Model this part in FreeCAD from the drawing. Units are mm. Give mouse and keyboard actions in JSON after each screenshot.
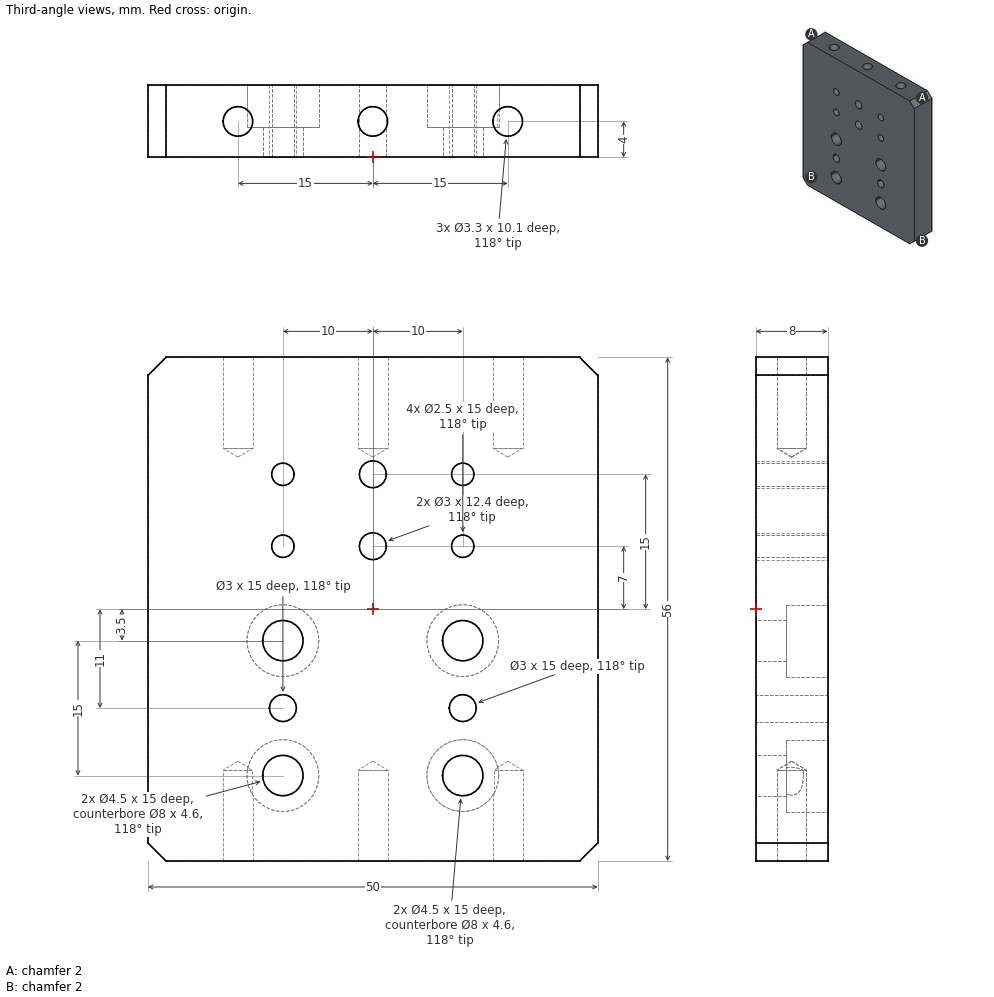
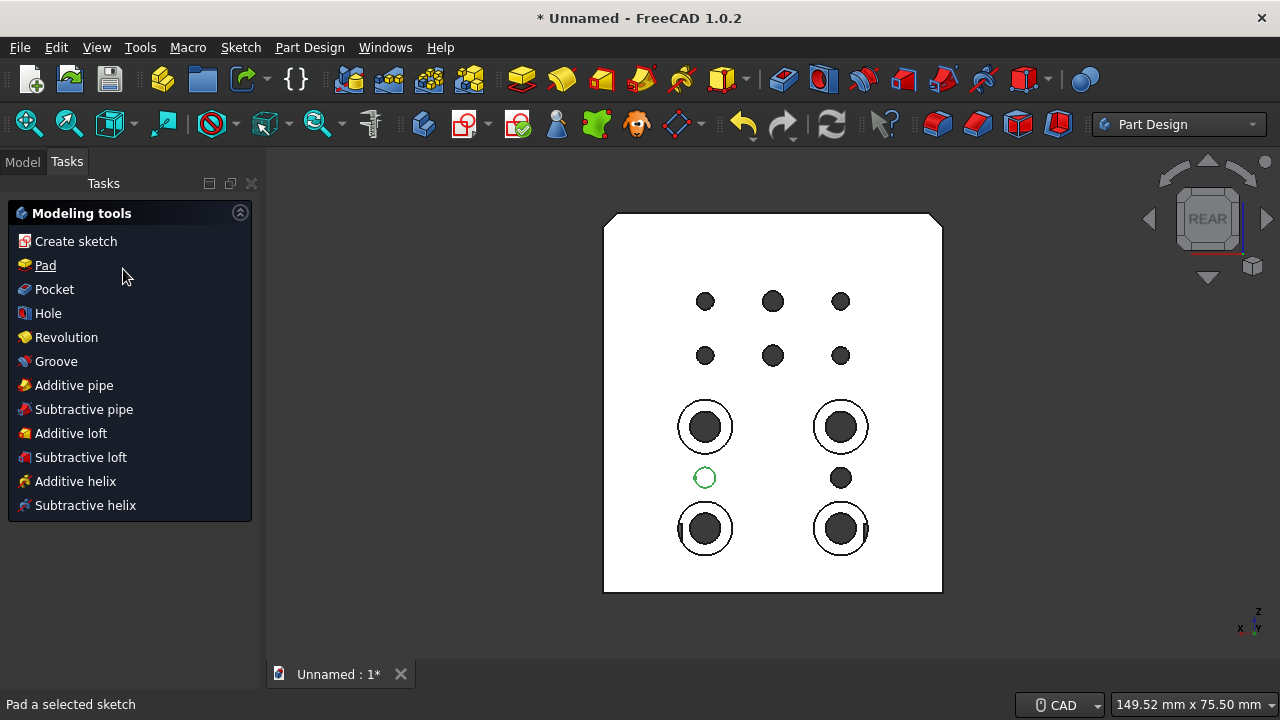
{"action": "left_click", "coordinate": [824, 80]}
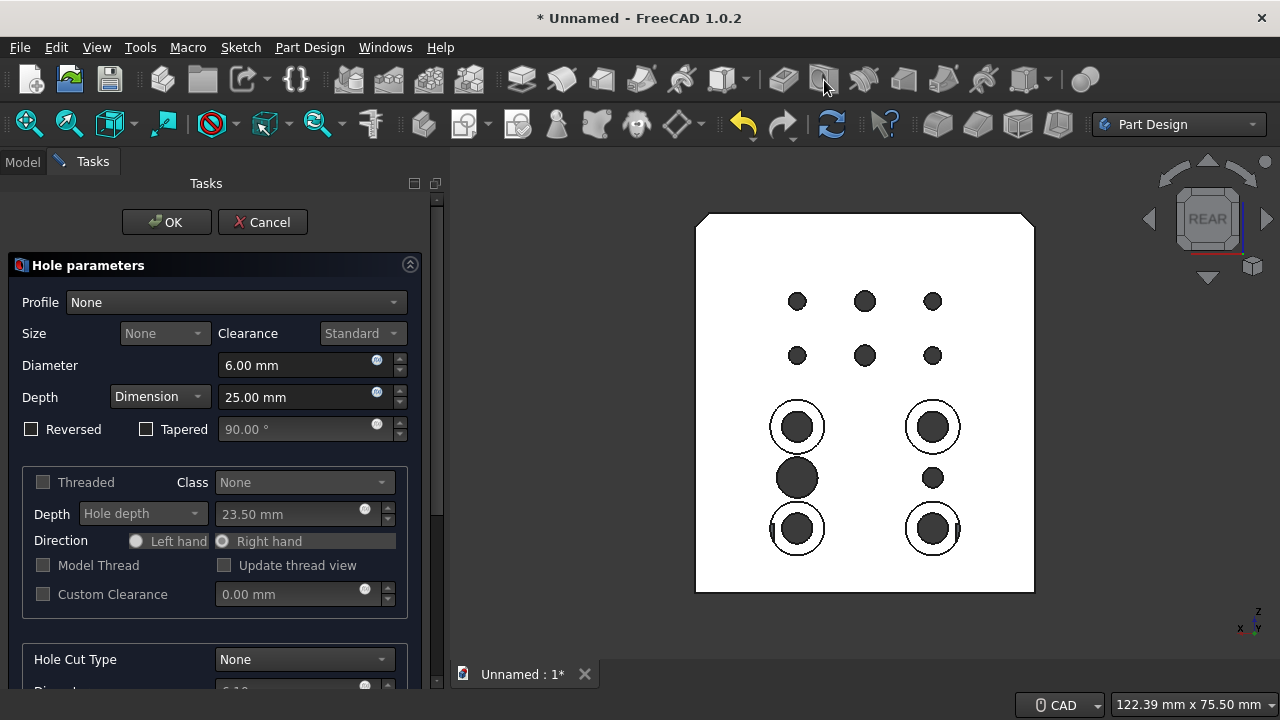
{"action": "triple_click", "coordinate": [305, 365]}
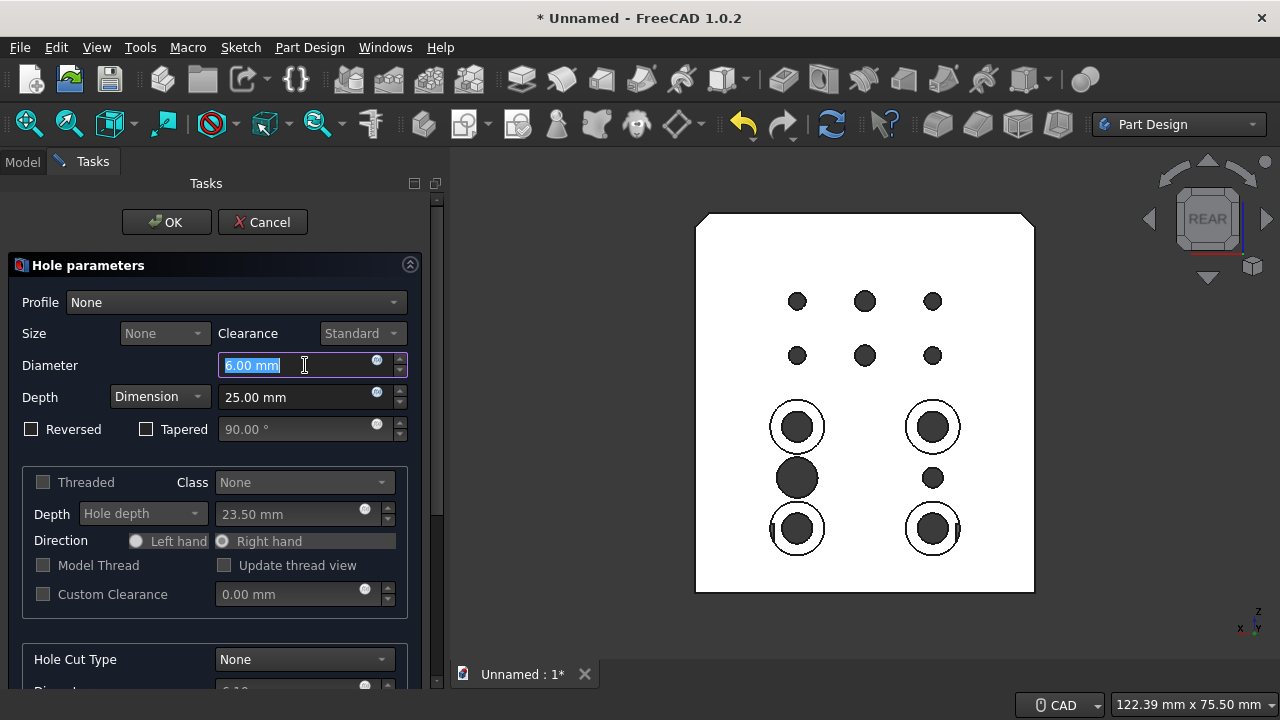
{"action": "type", "text": "3"}
{"action": "key", "text": "Tab"}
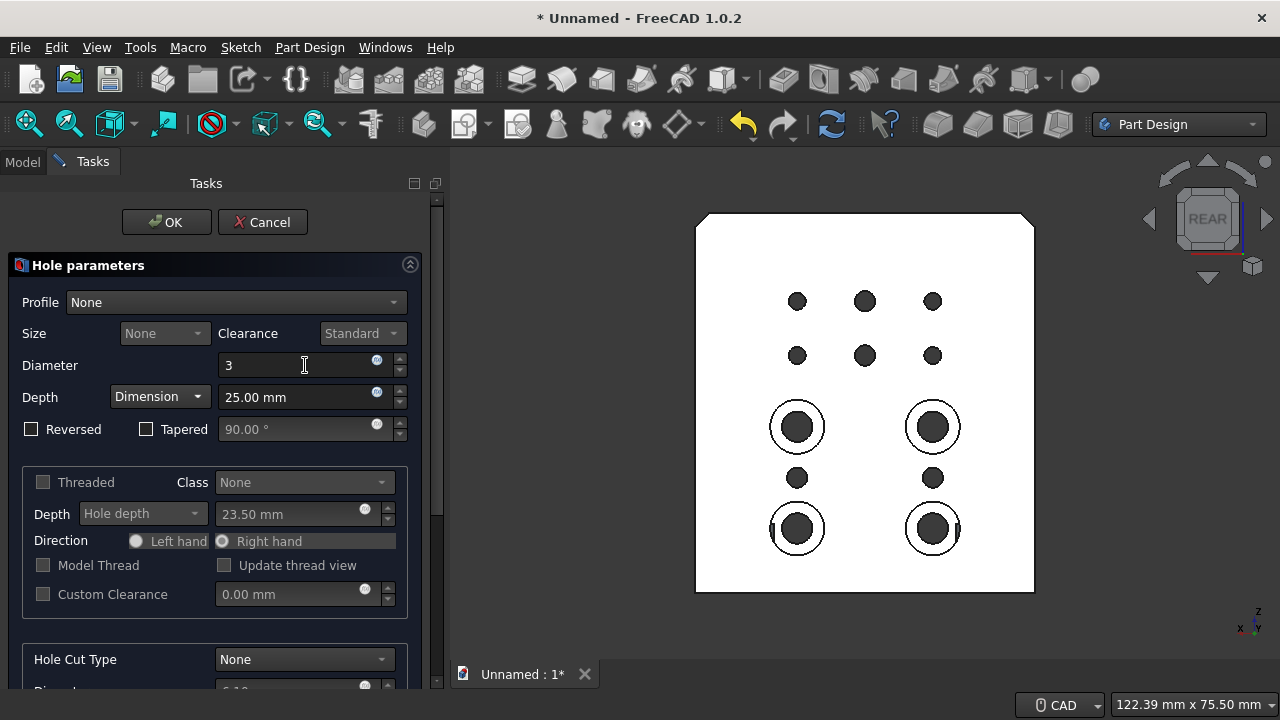
{"action": "triple_click", "coordinate": [305, 397]}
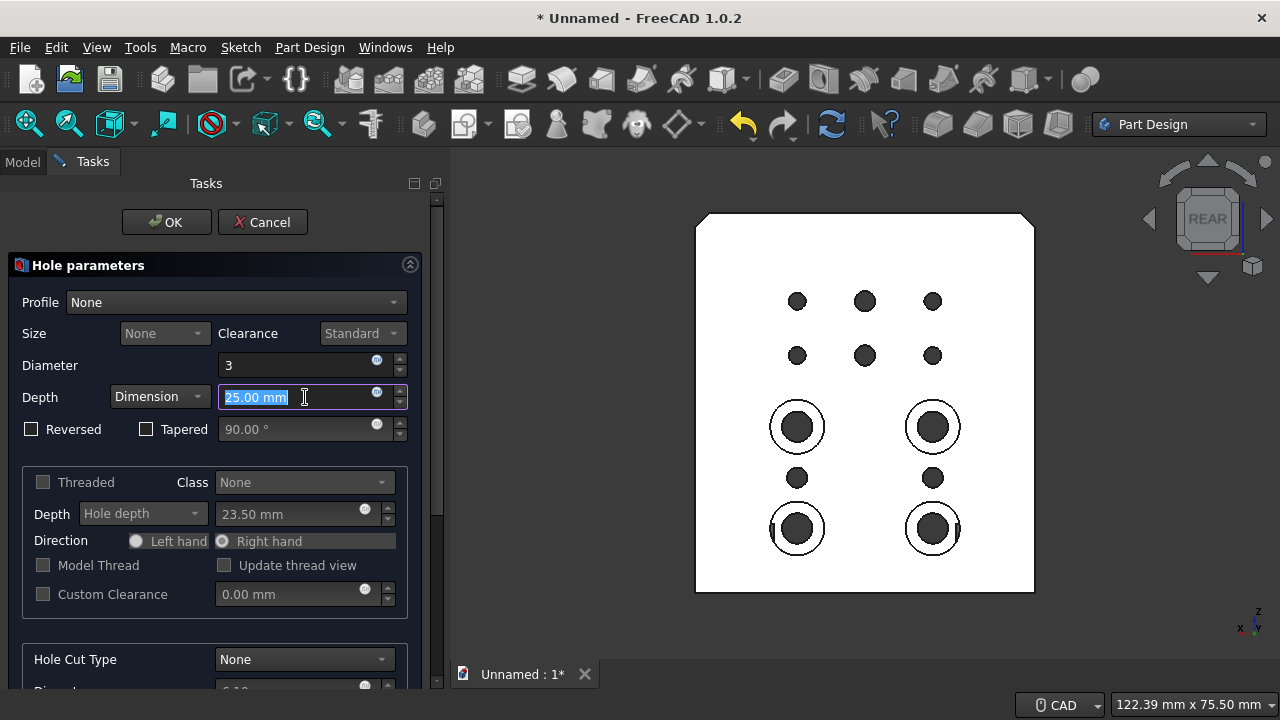
{"action": "type", "text": "15"}
{"action": "key", "text": "Tab"}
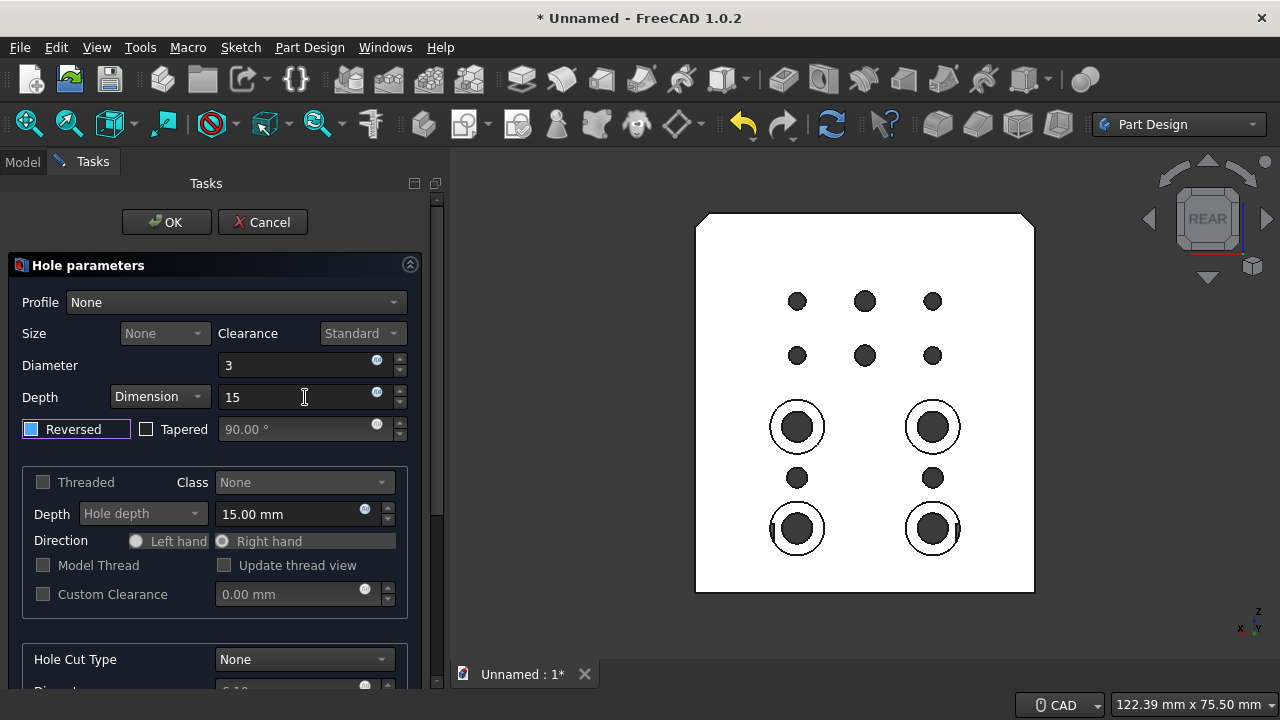
{"action": "left_click", "coordinate": [167, 222]}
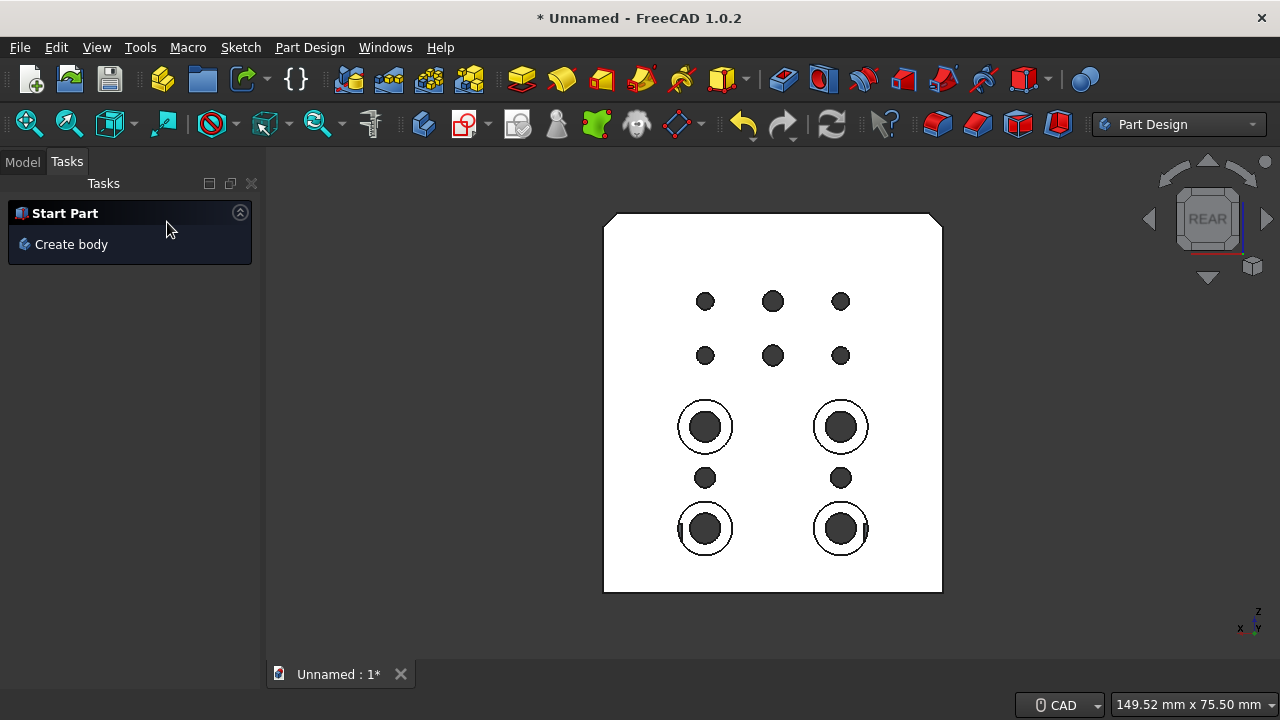
{"action": "key", "text": "0"}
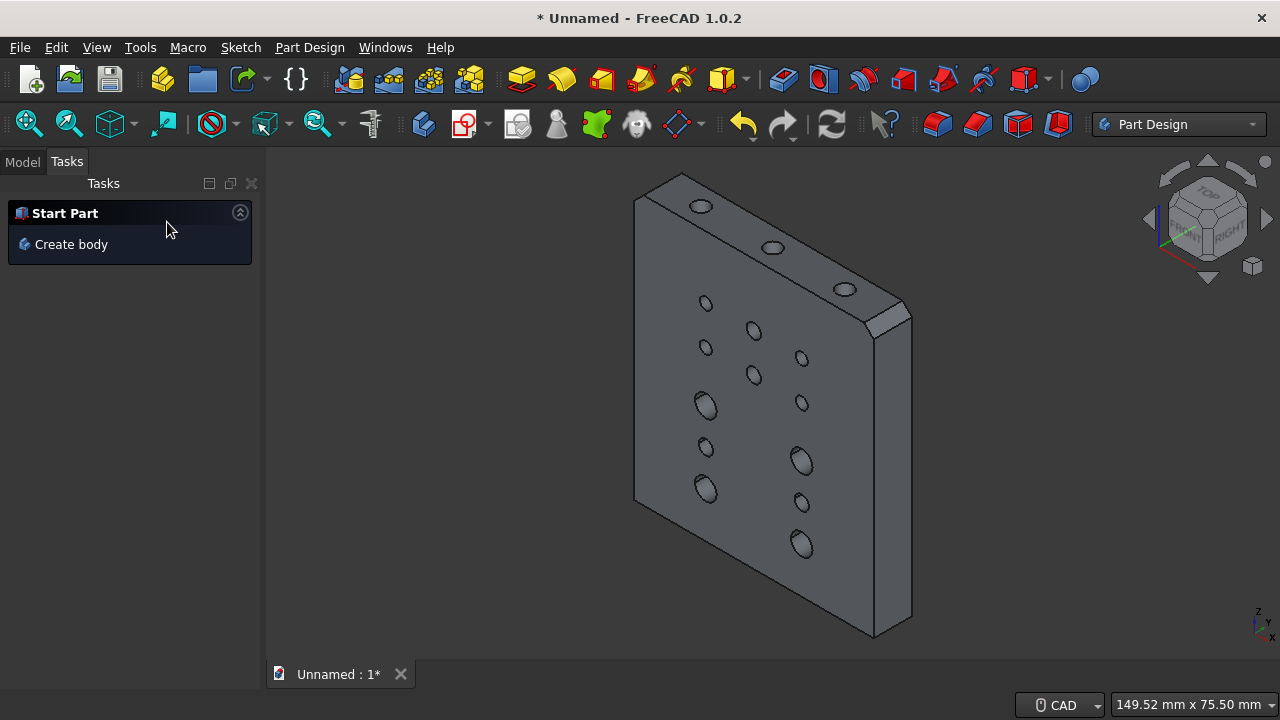
{"action": "key", "text": "2"}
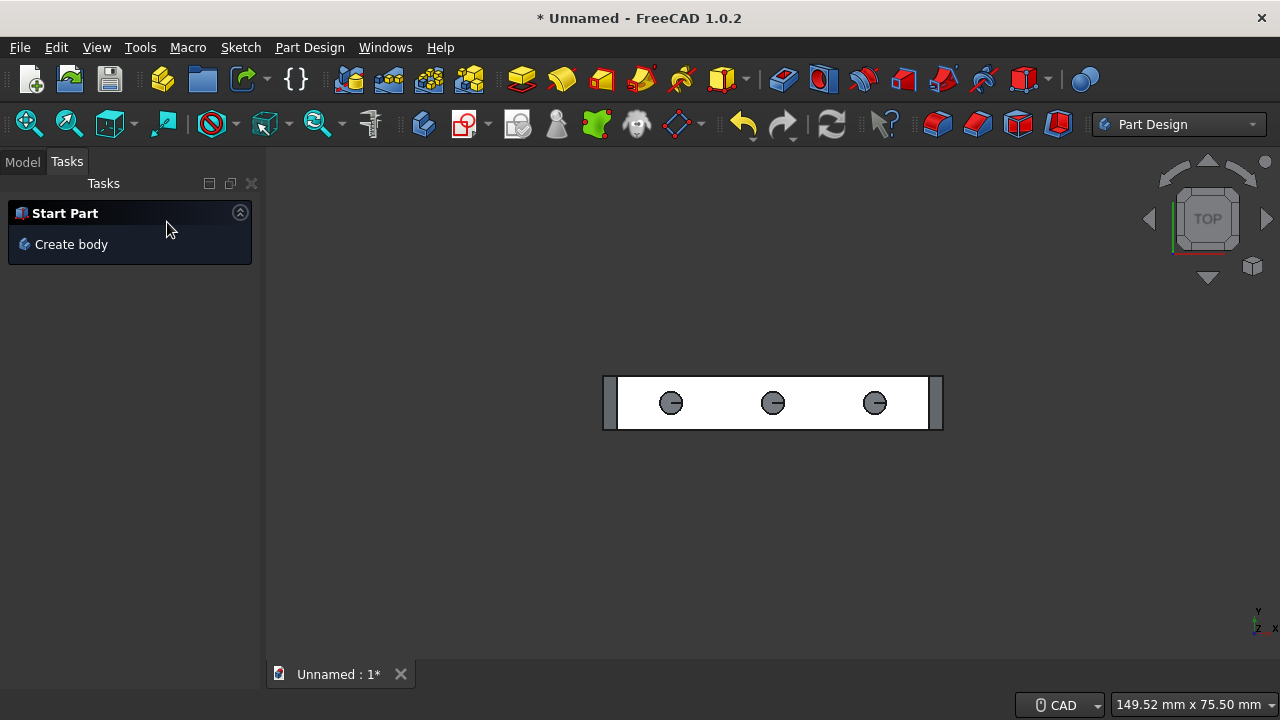
{"action": "key", "text": "v f"}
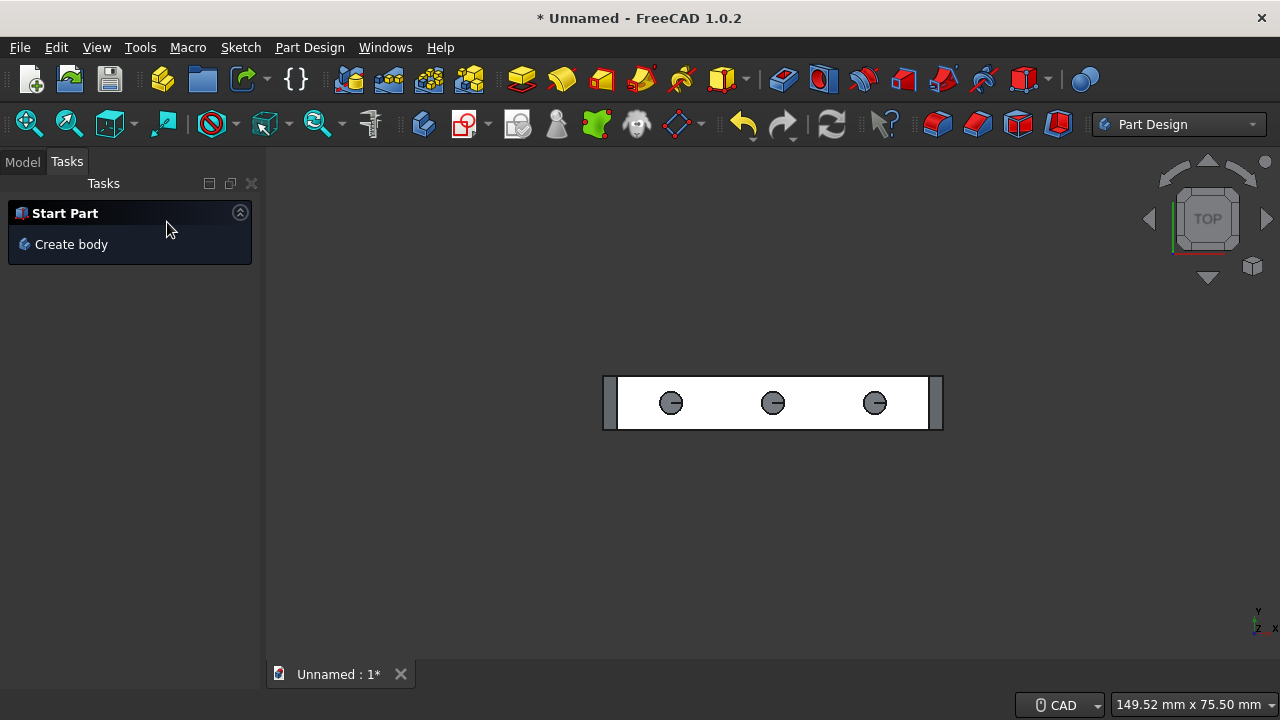
{"action": "key", "text": "1"}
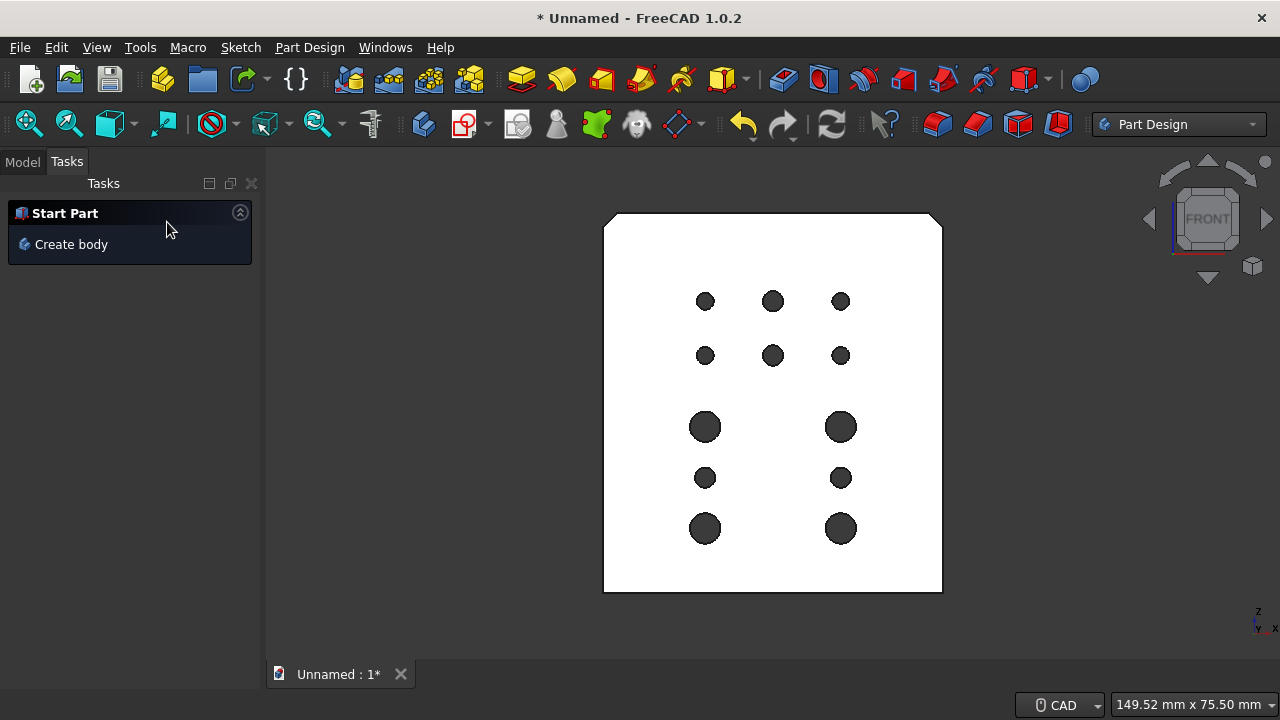
{"action": "key", "text": "3"}